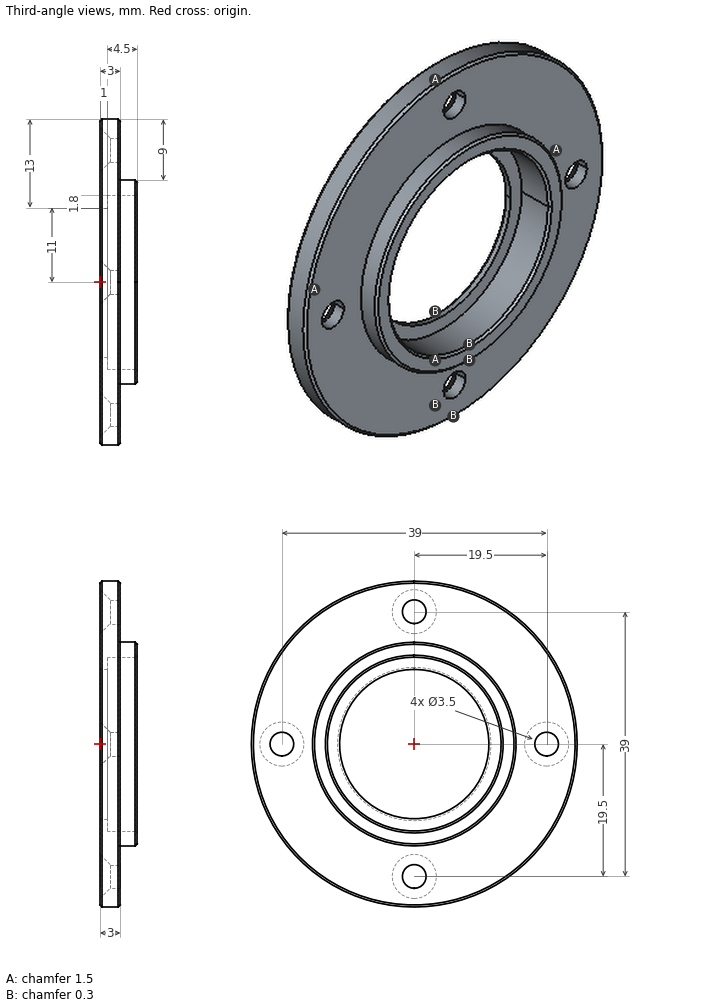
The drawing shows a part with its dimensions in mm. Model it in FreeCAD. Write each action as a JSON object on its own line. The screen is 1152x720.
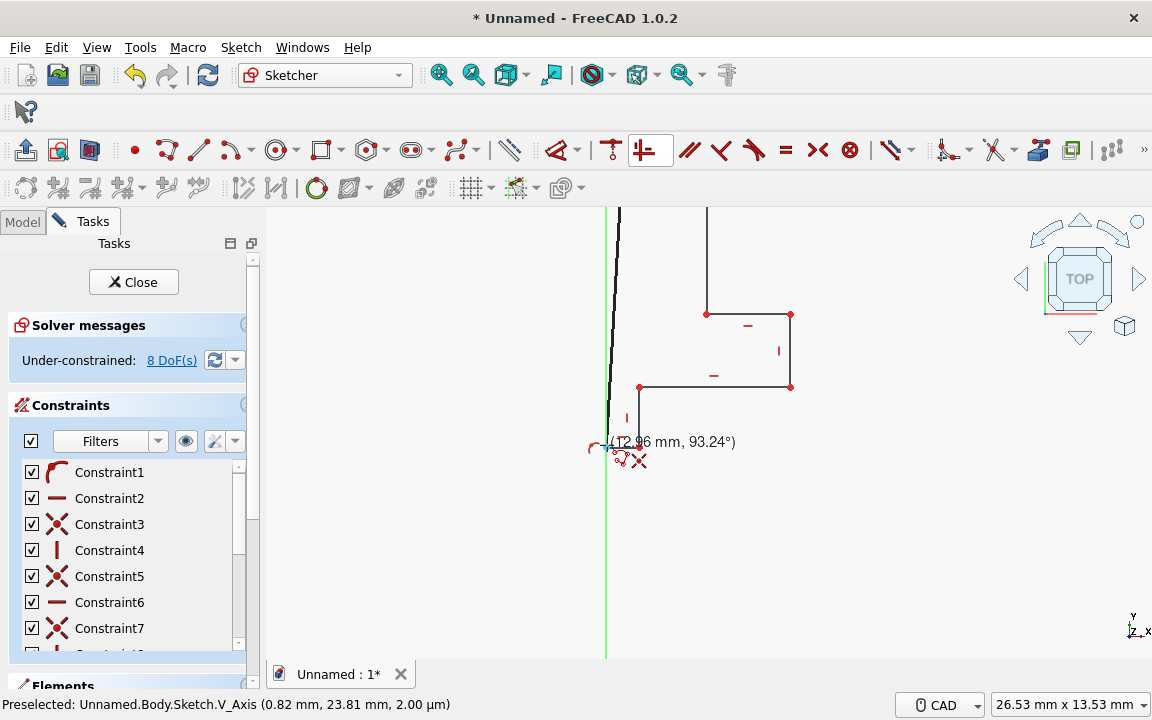
{"action": "left_click", "coordinate": [606, 448]}
{"action": "key", "text": "Escape"}
{"action": "key", "text": "Escape"}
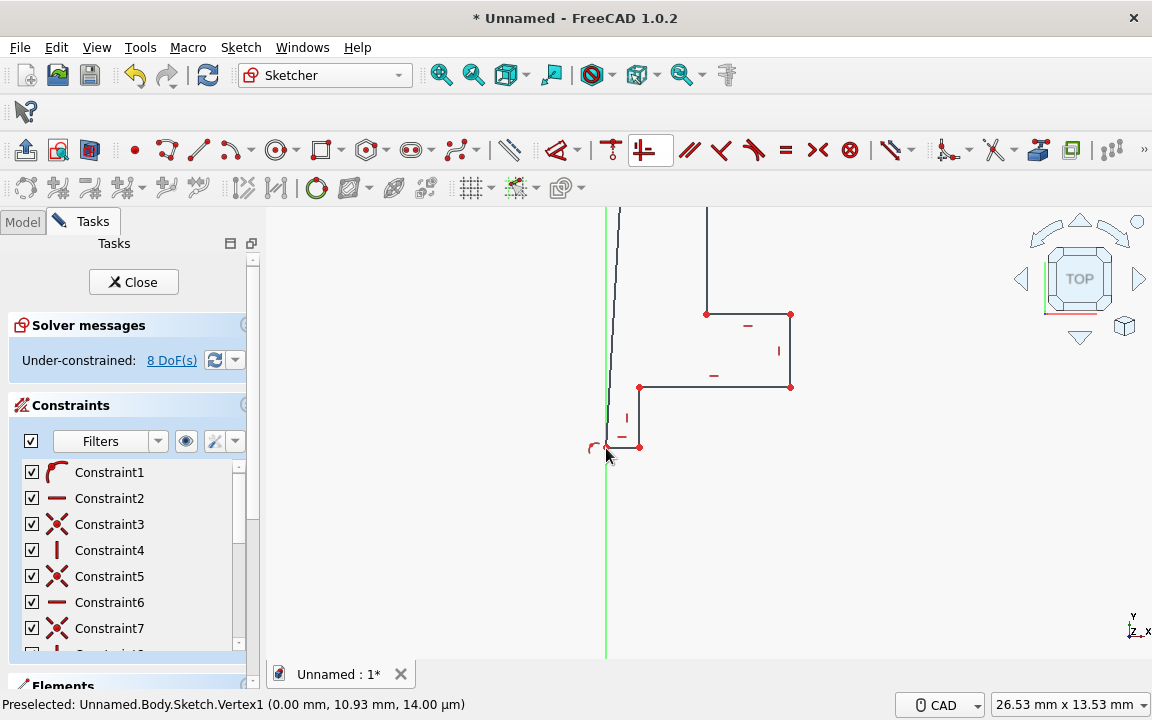
{"action": "scroll", "coordinate": [616, 274], "scroll_direction": "up", "scroll_amount": 2}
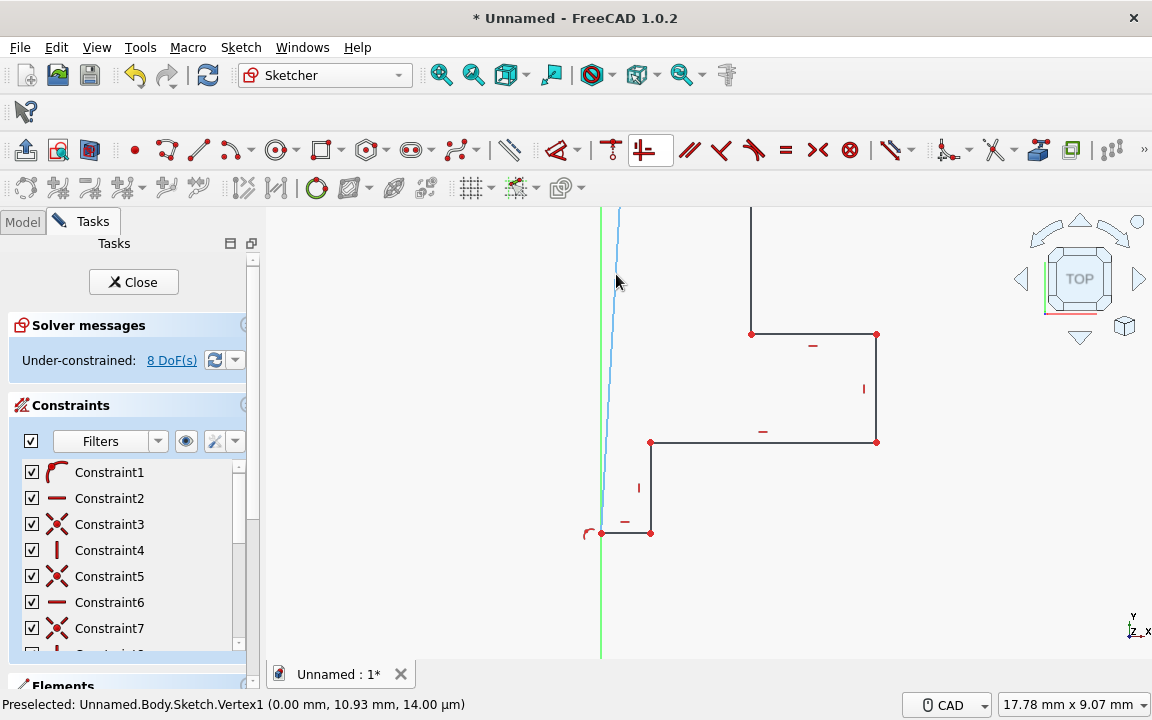
{"action": "left_click", "coordinate": [616, 275]}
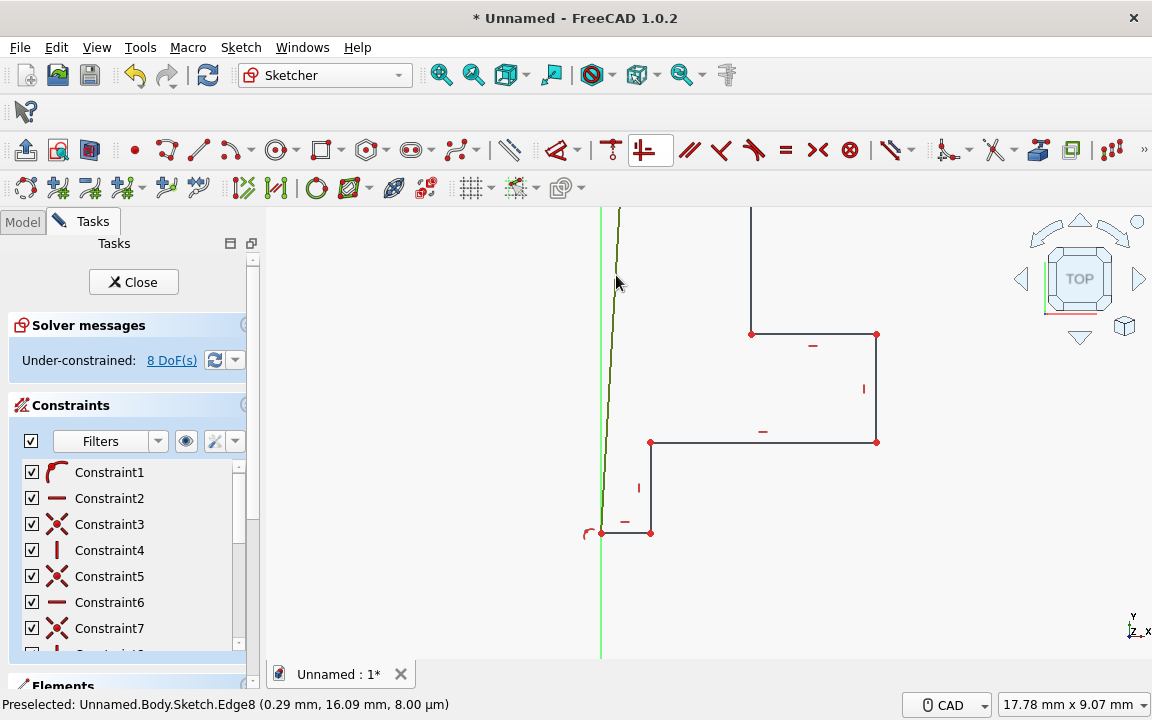
{"action": "key", "text": "v"}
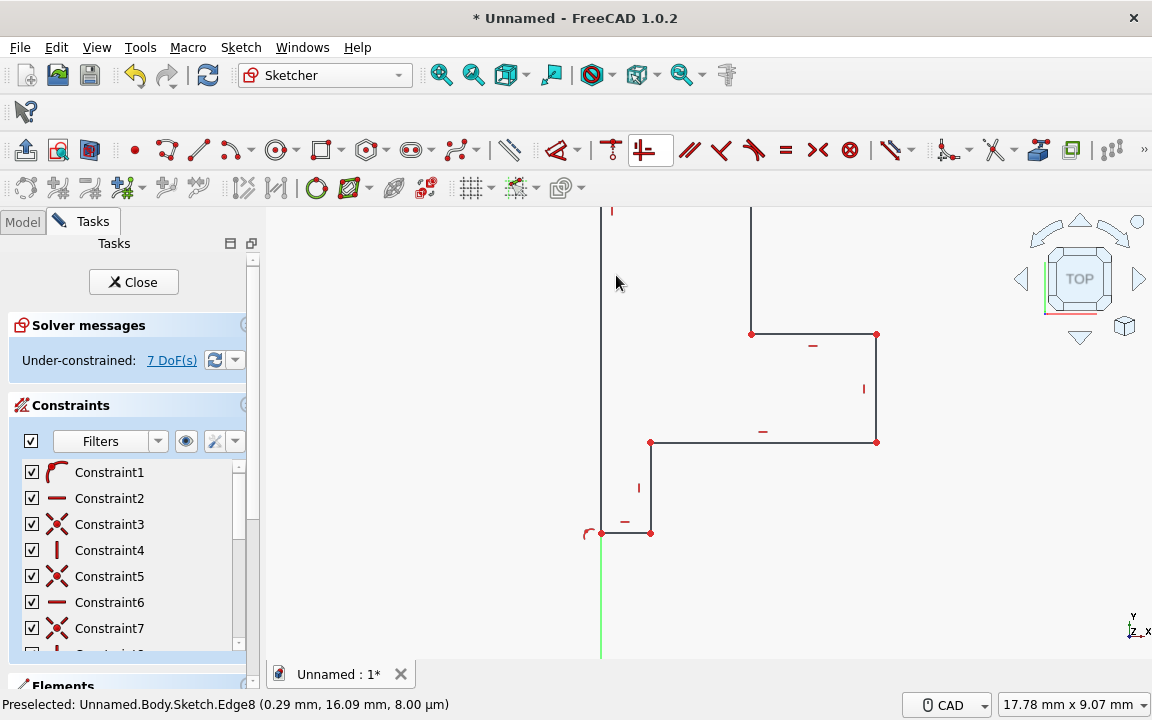
{"action": "left_click", "coordinate": [556, 150]}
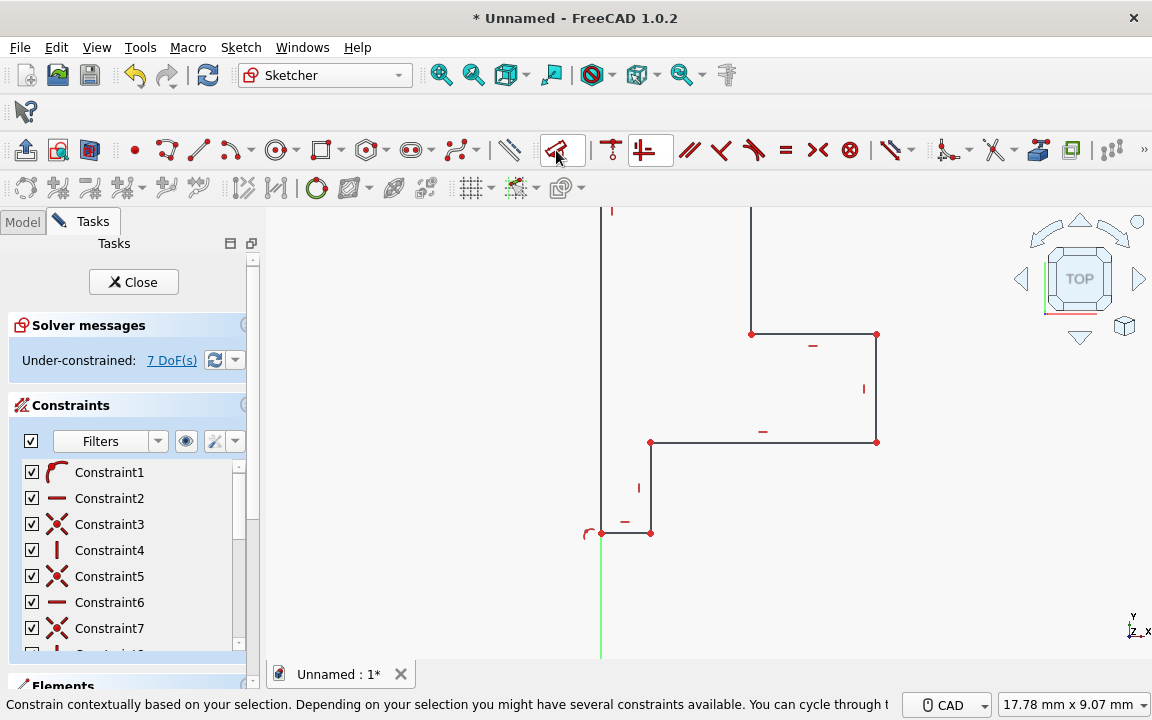
{"action": "left_click", "coordinate": [616, 533]}
{"action": "left_click", "coordinate": [626, 567]}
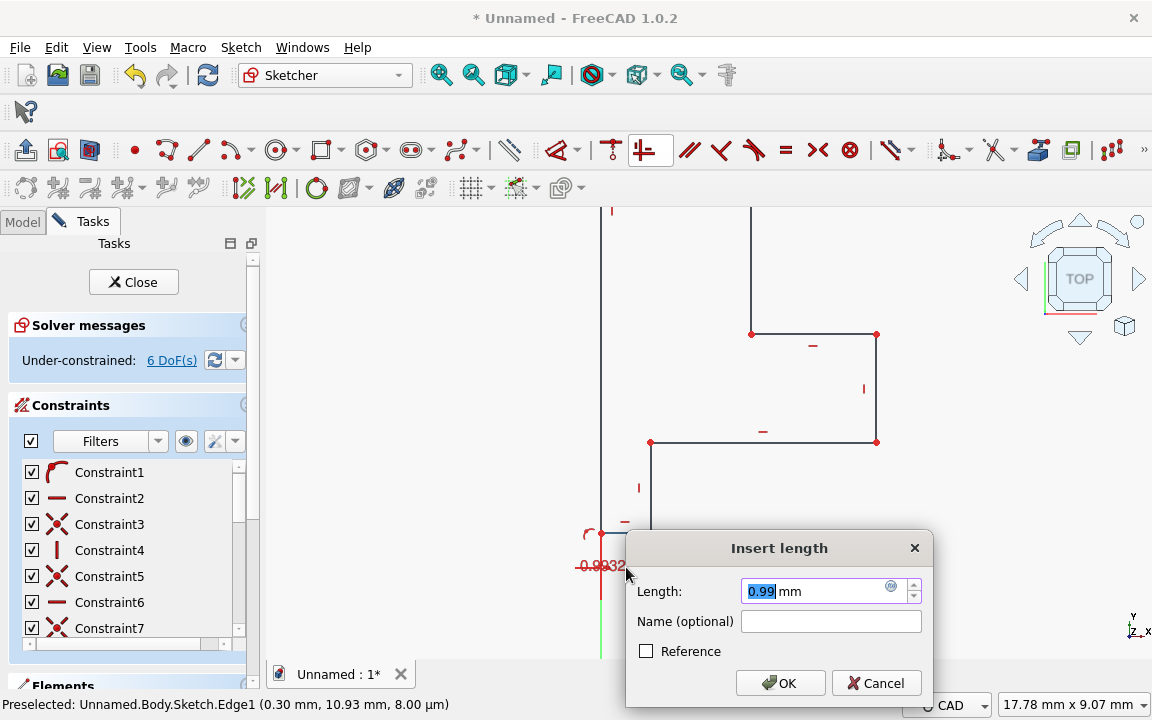
{"action": "type", "text": "1"}
{"action": "key", "text": "Return"}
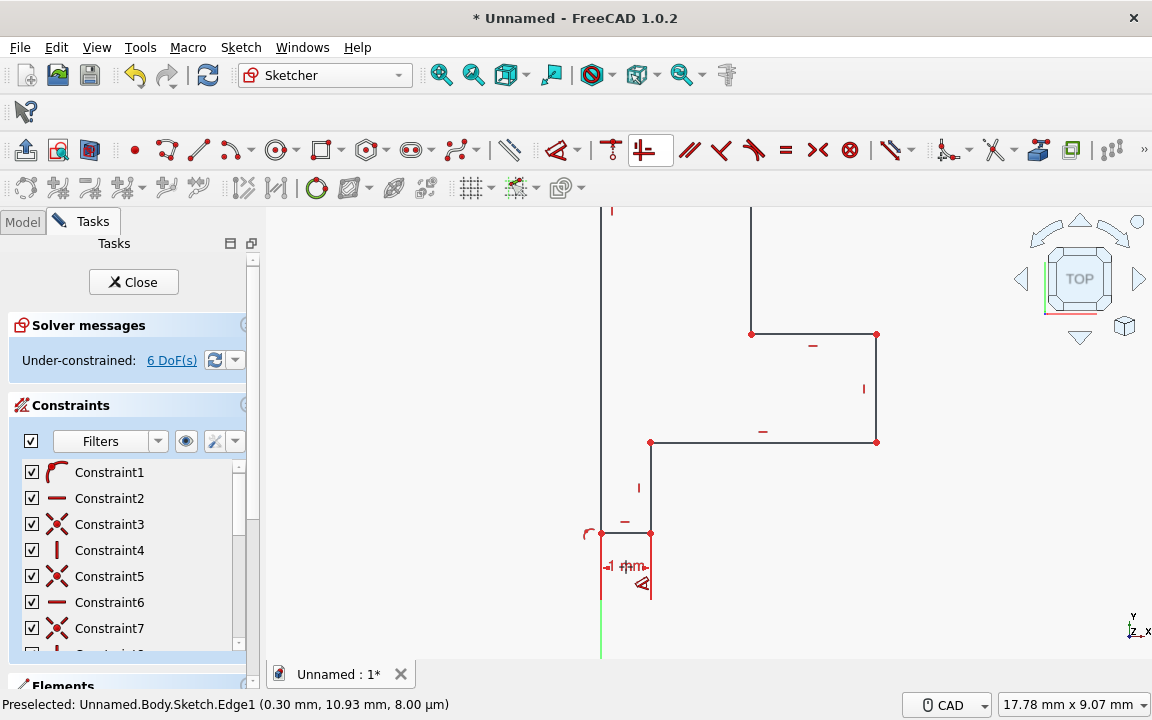
{"action": "scroll", "coordinate": [609, 418], "scroll_direction": "down", "scroll_amount": 7}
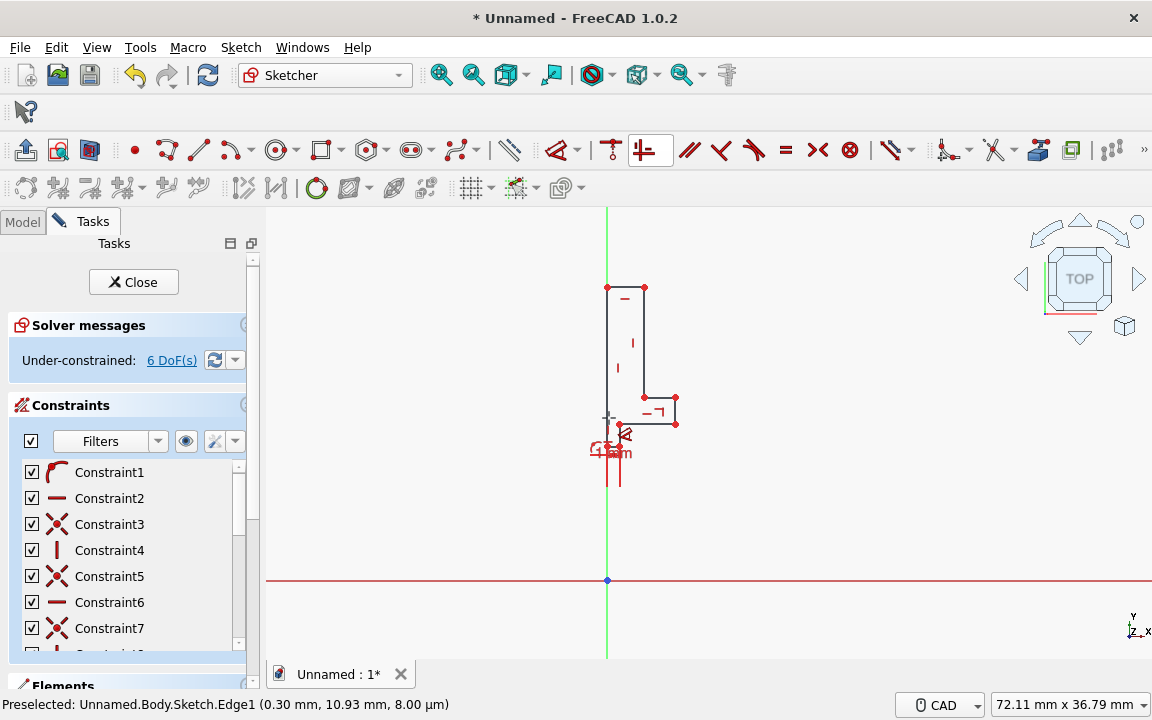
{"action": "left_click", "coordinate": [644, 376]}
{"action": "left_click", "coordinate": [678, 343]}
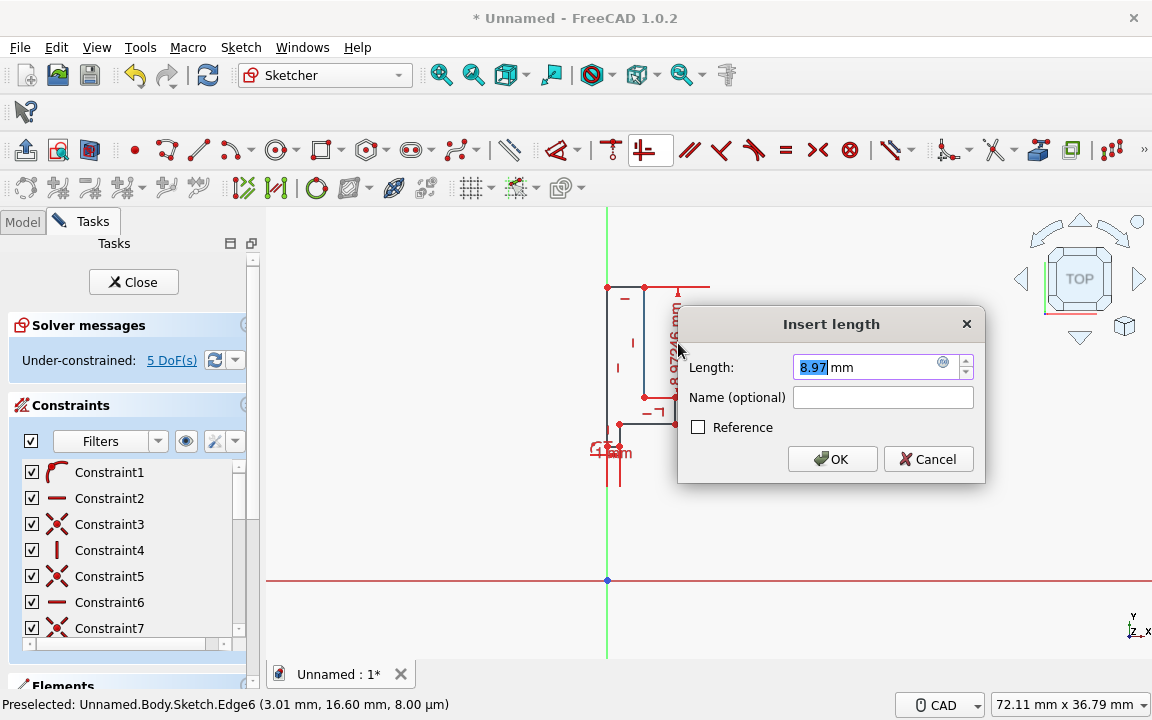
{"action": "type", "text": "9"}
{"action": "key", "text": "Return"}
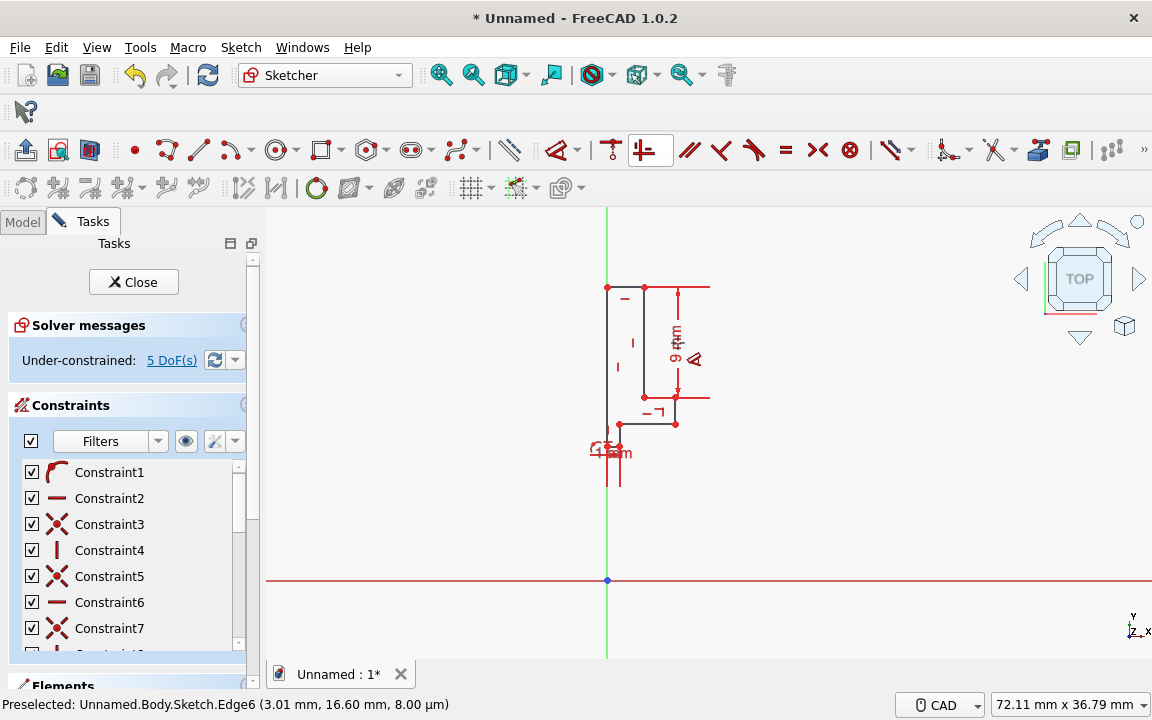
{"action": "scroll", "coordinate": [633, 287], "scroll_direction": "up", "scroll_amount": 2}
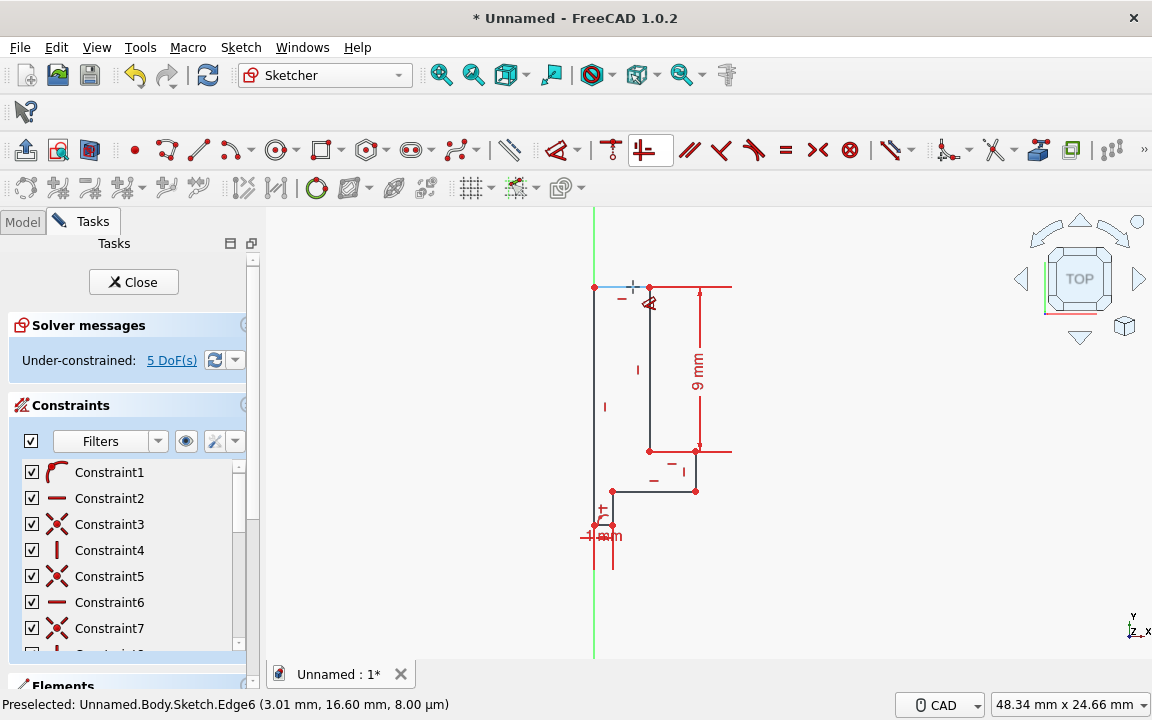
{"action": "left_click", "coordinate": [633, 287]}
{"action": "left_click", "coordinate": [622, 253]}